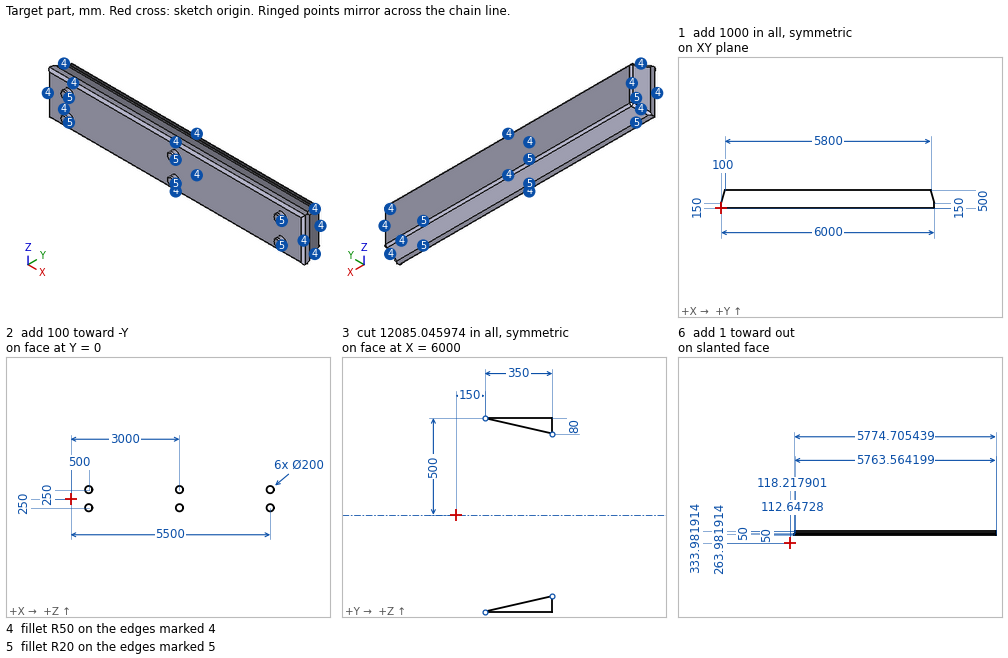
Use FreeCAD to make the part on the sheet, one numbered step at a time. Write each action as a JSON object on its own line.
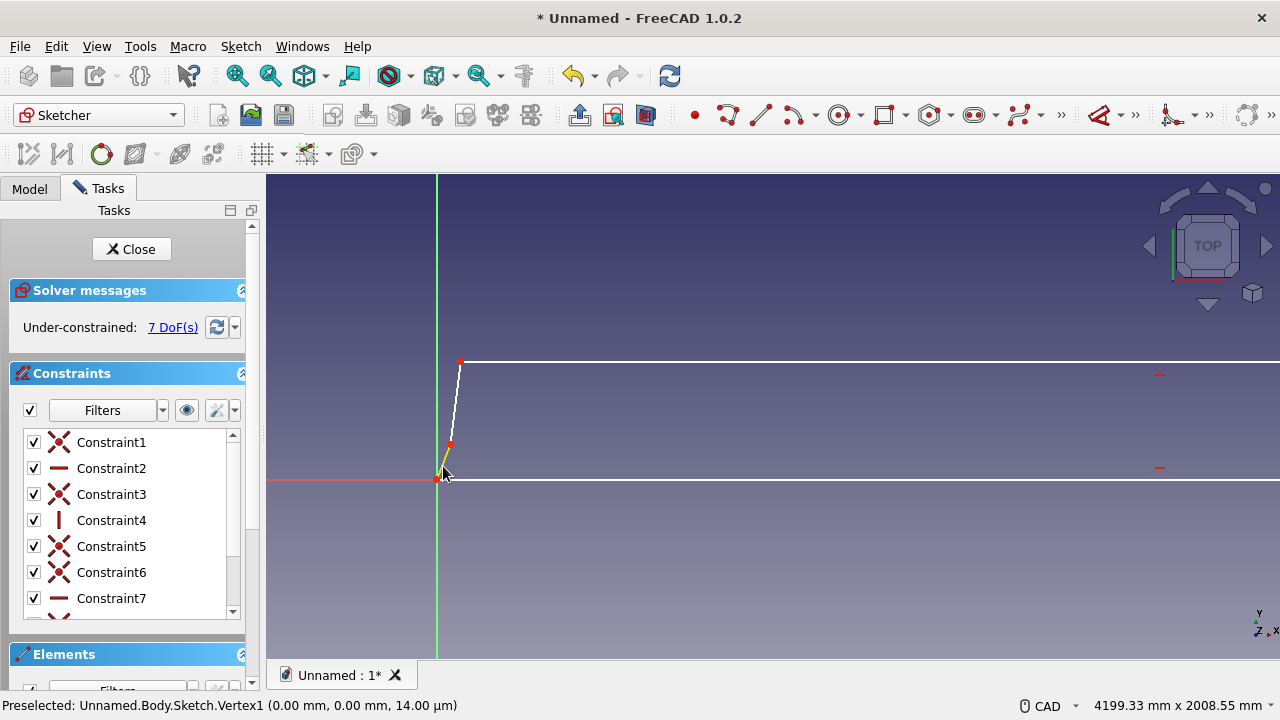
{"action": "left_click", "coordinate": [442, 466]}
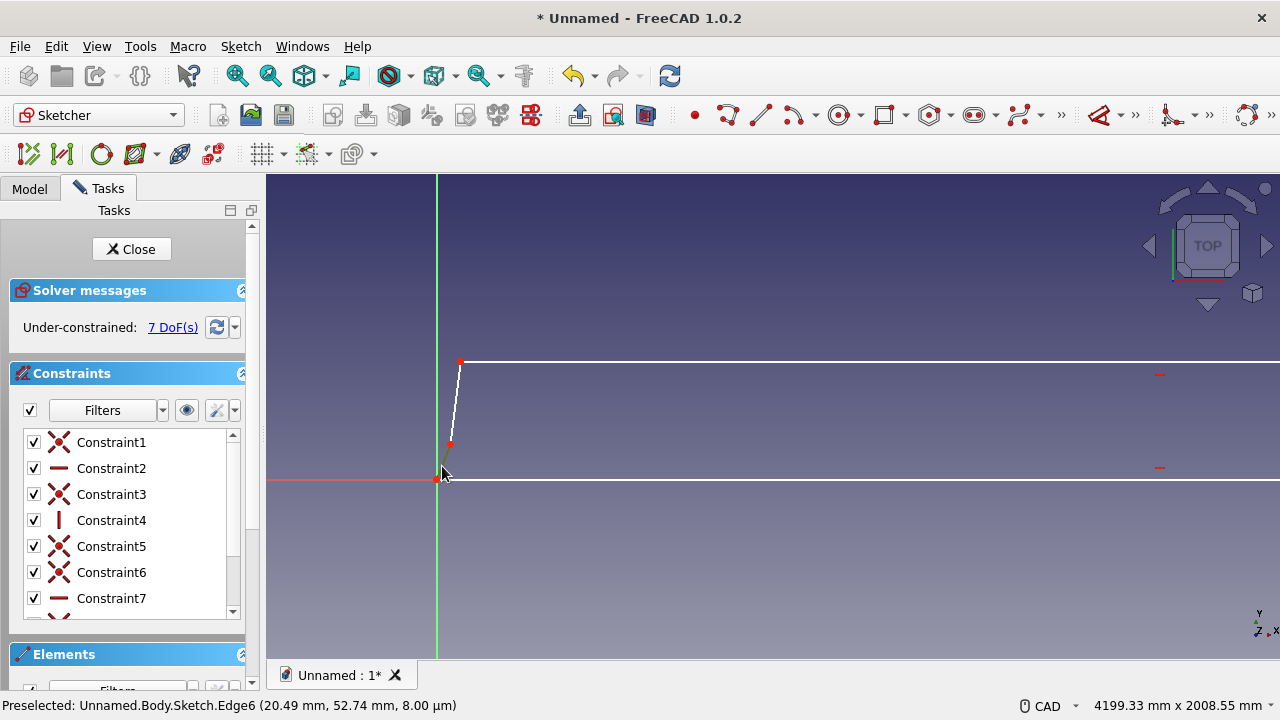
{"action": "key", "text": "v"}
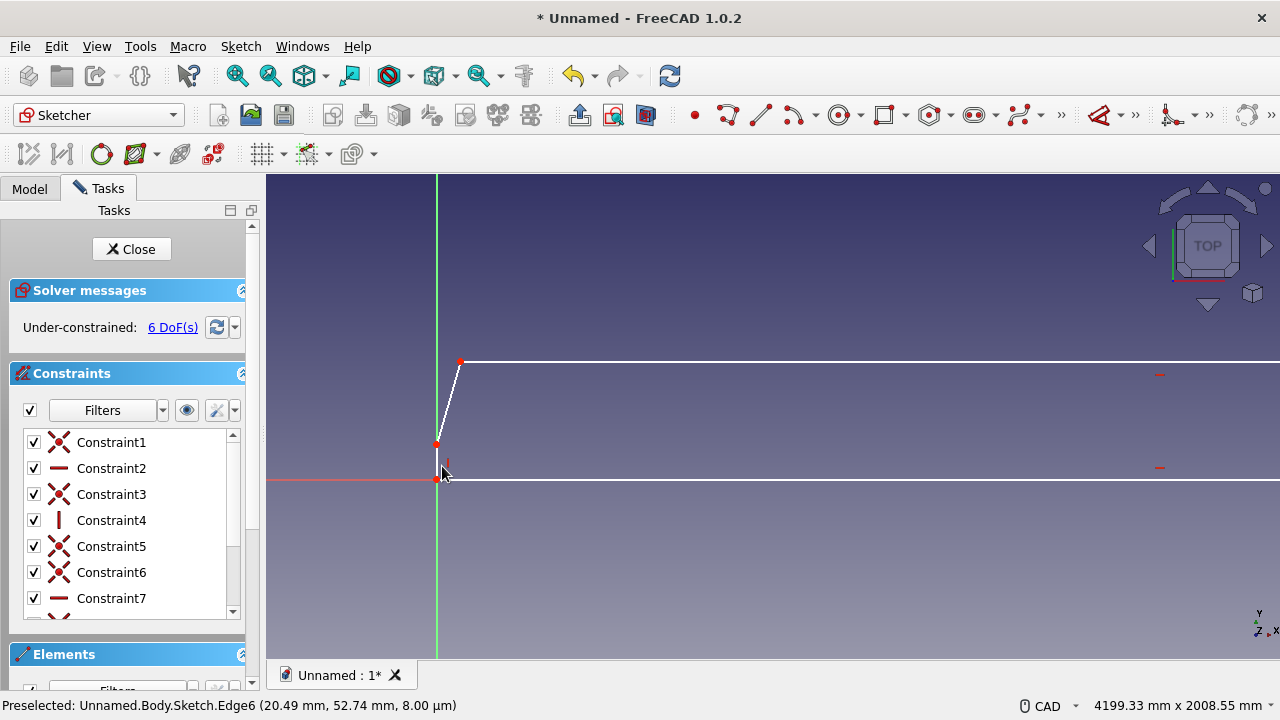
{"action": "scroll", "coordinate": [439, 415], "scroll_direction": "down", "scroll_amount": 5}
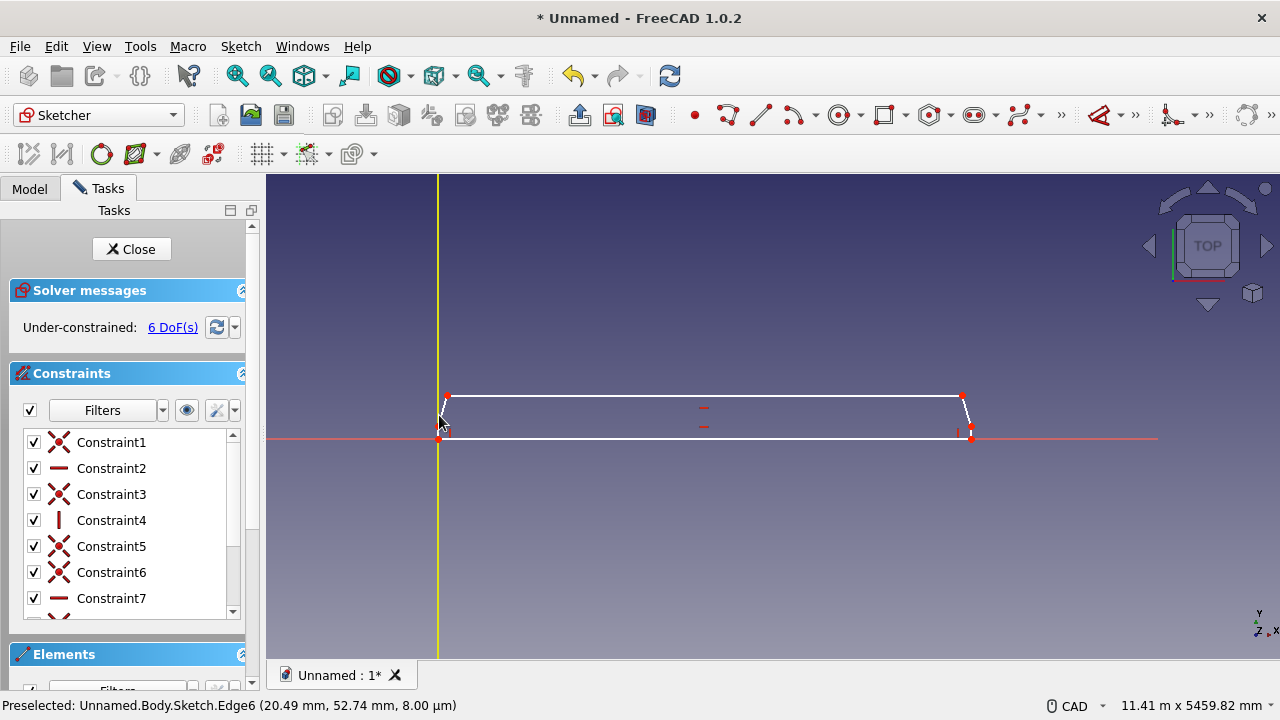
{"action": "scroll", "coordinate": [971, 435], "scroll_direction": "up", "scroll_amount": 7}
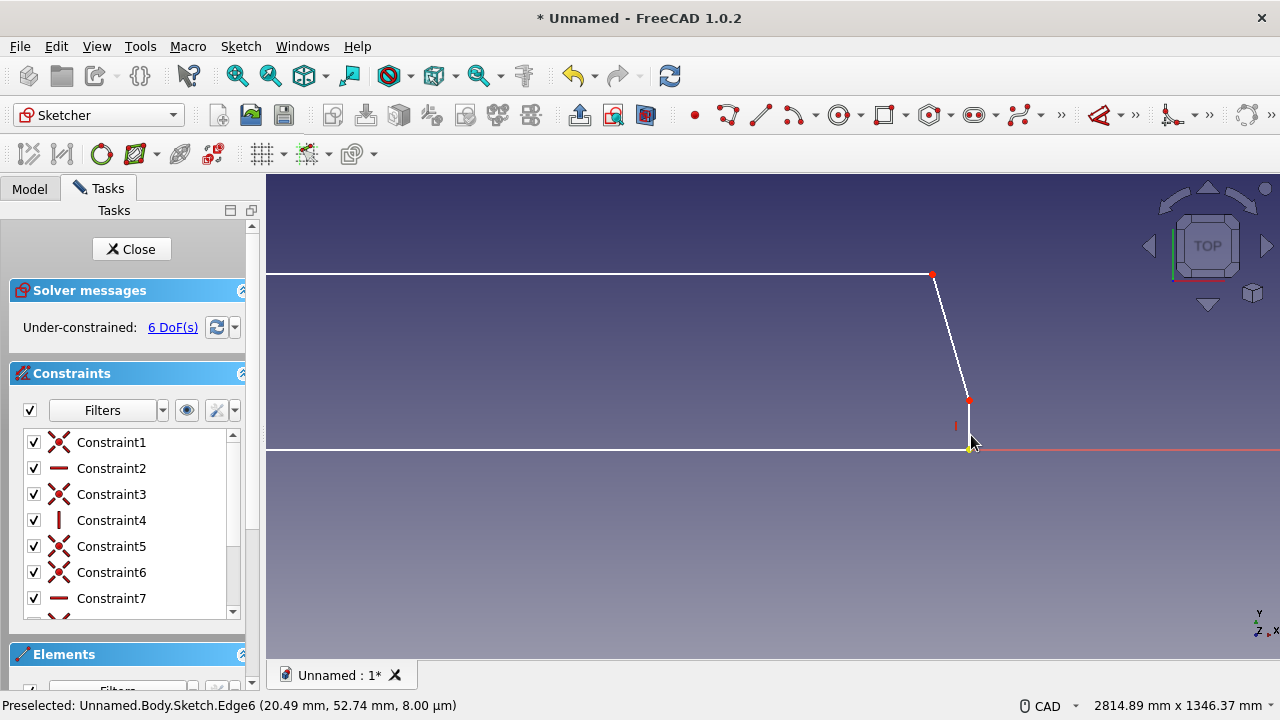
{"action": "left_click", "coordinate": [969, 435]}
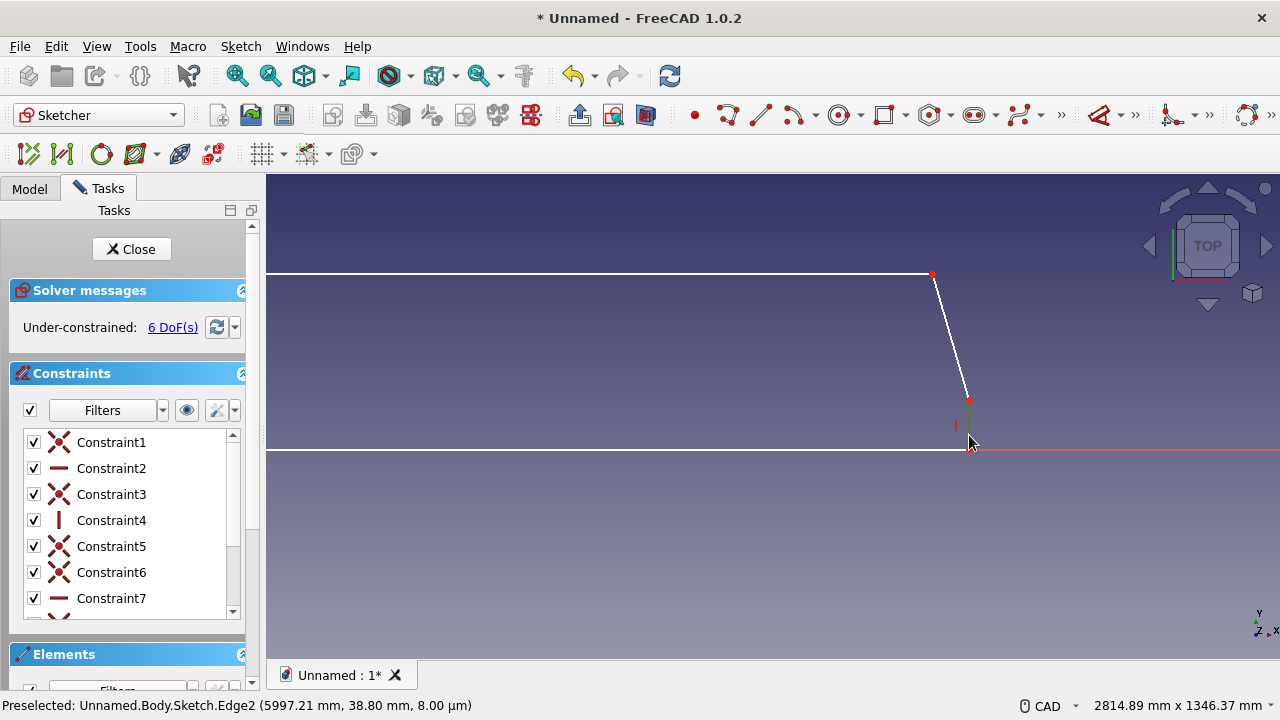
{"action": "key", "text": "i"}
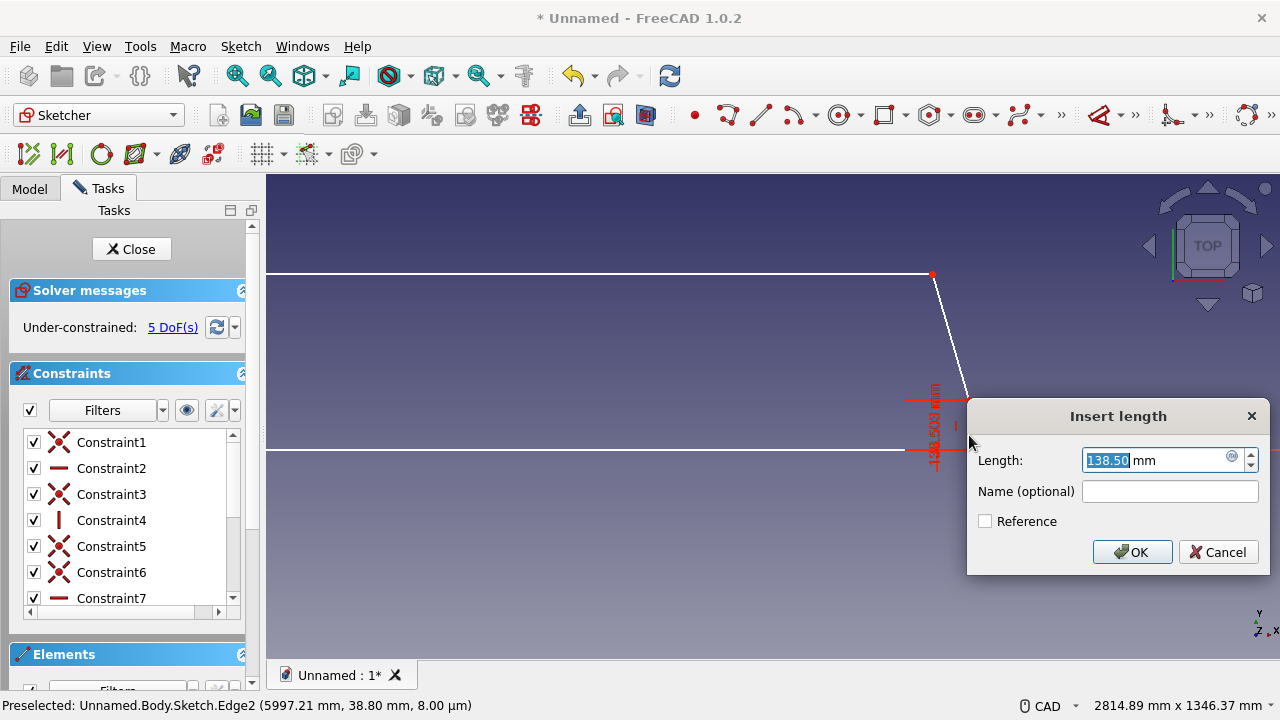
{"action": "type", "text": "150"}
{"action": "key", "text": "Return"}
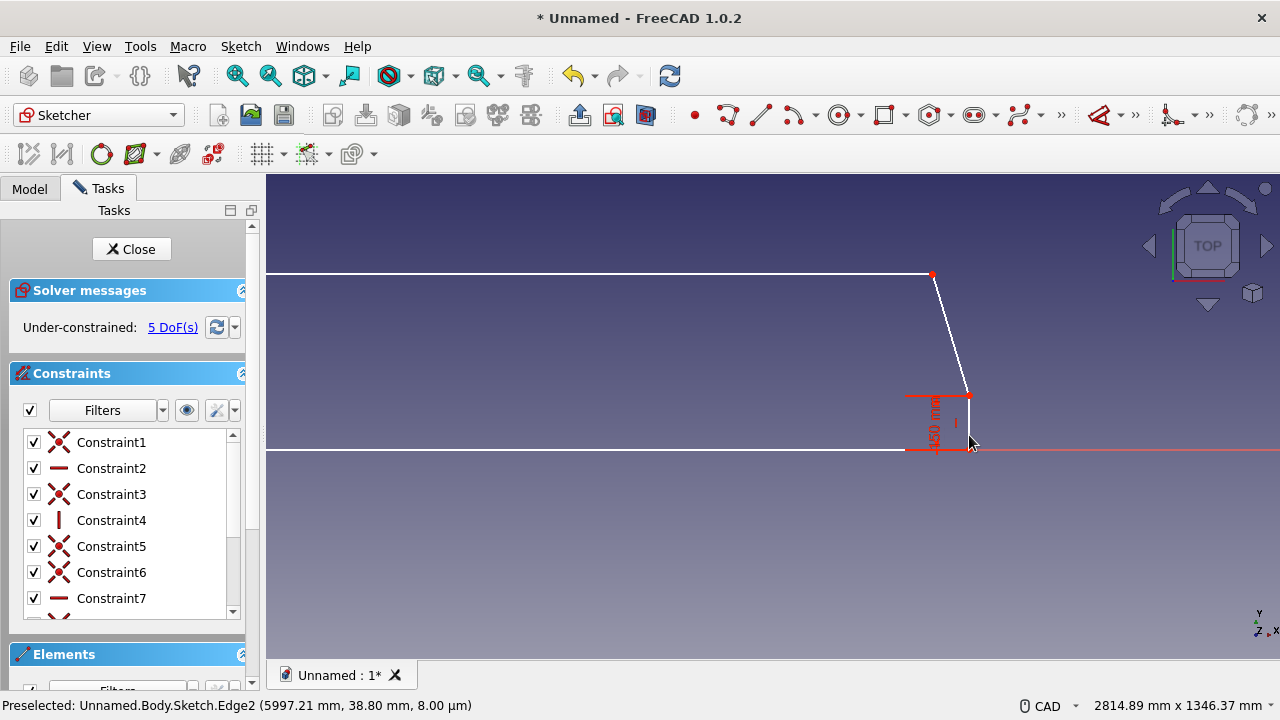
{"action": "scroll", "coordinate": [971, 435], "scroll_direction": "down", "scroll_amount": 7}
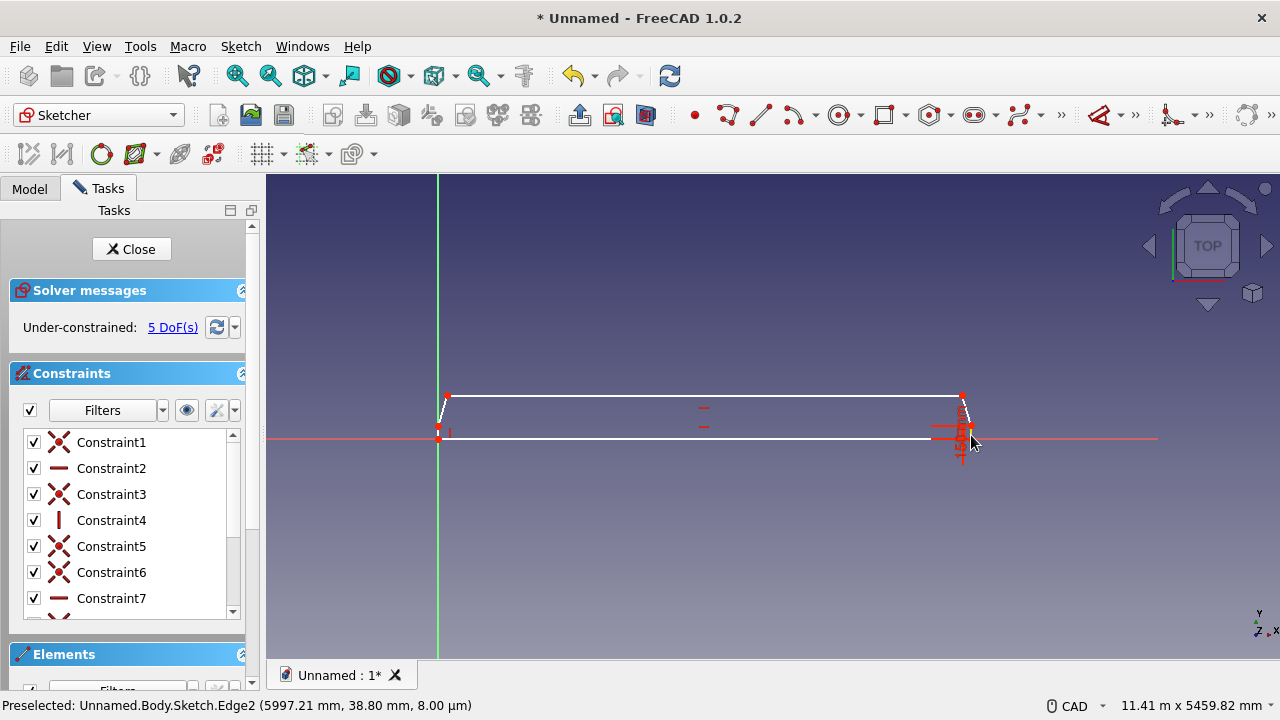
{"action": "scroll", "coordinate": [438, 430], "scroll_direction": "up", "scroll_amount": 7}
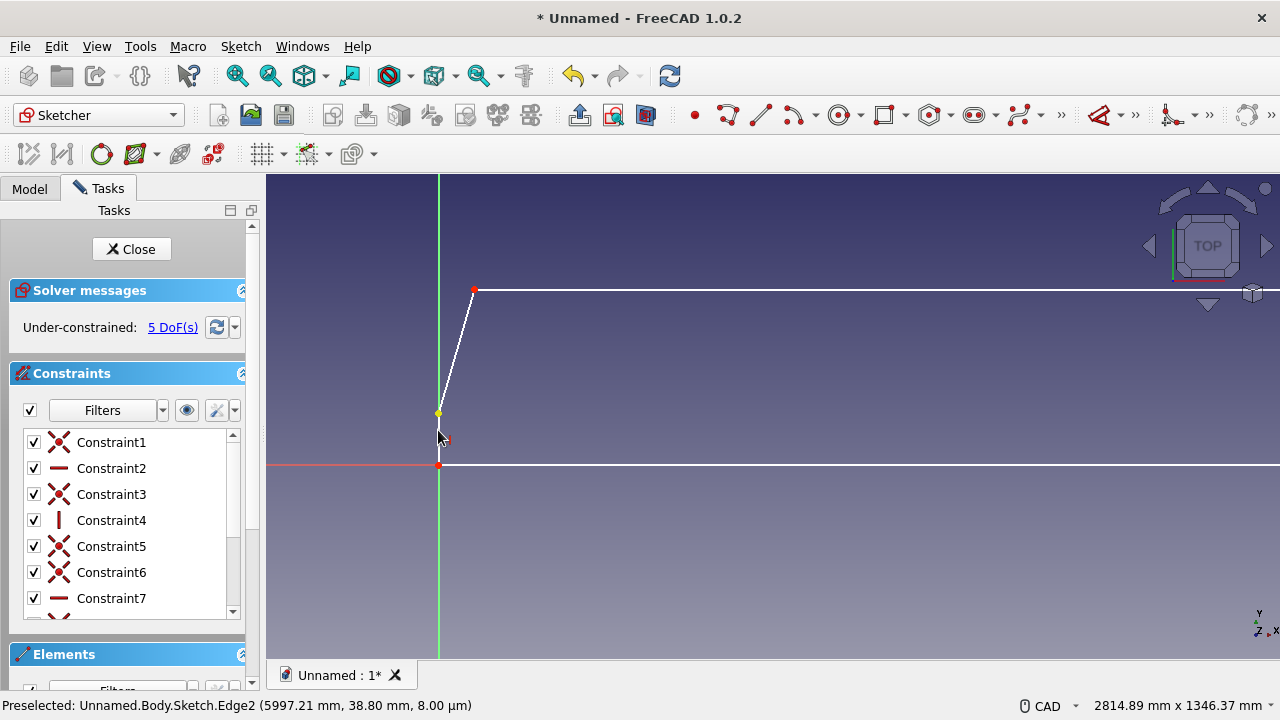
{"action": "left_click", "coordinate": [439, 429]}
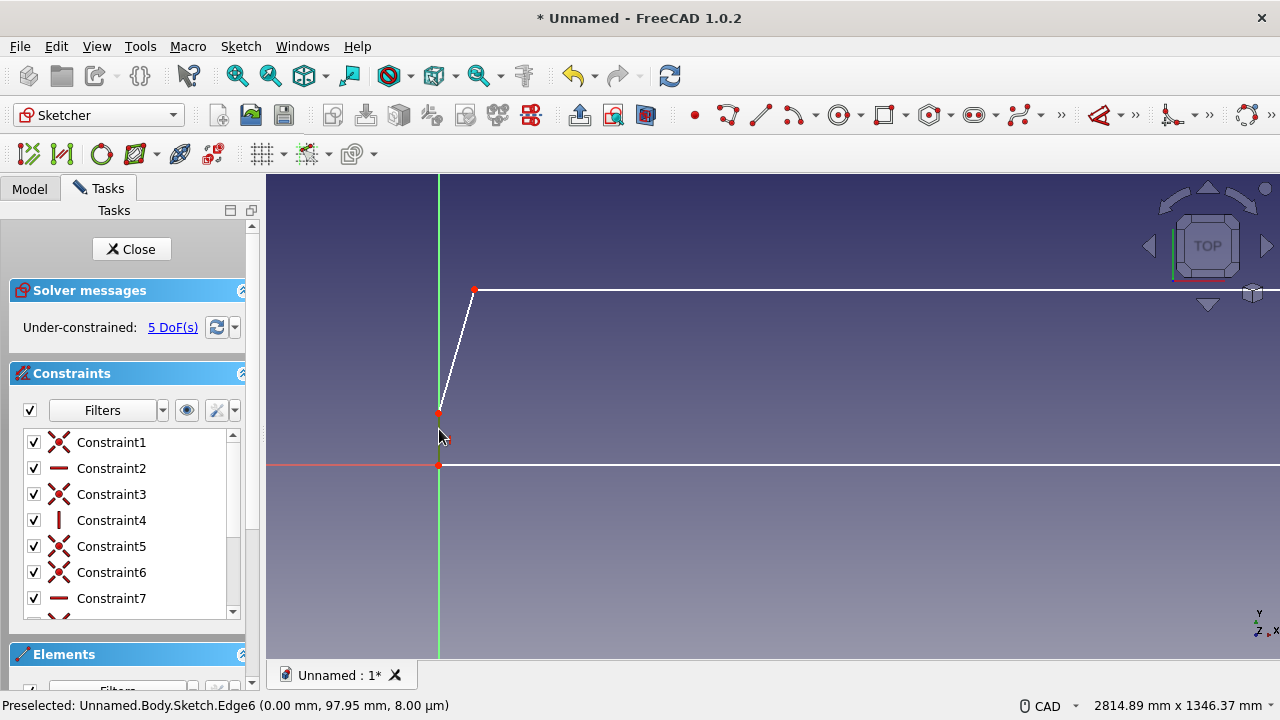
{"action": "key", "text": "i"}